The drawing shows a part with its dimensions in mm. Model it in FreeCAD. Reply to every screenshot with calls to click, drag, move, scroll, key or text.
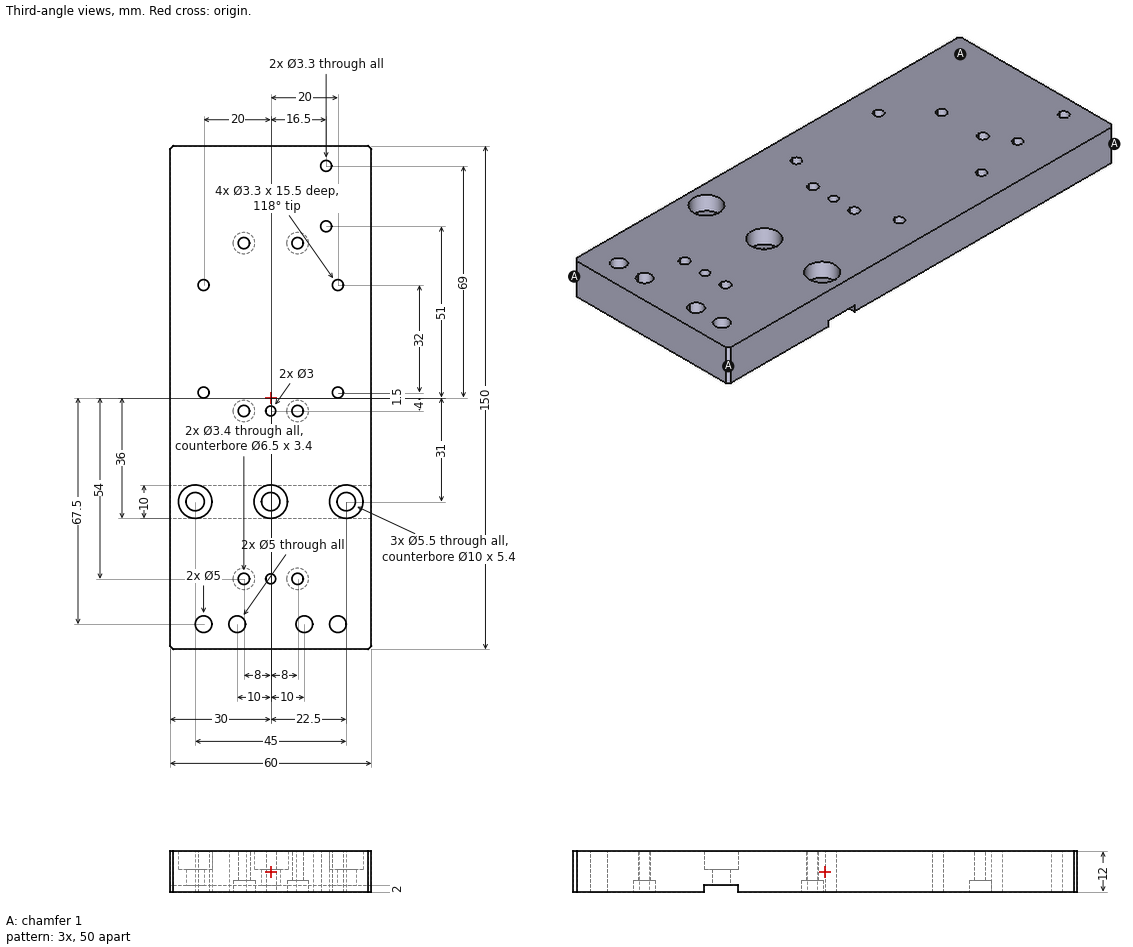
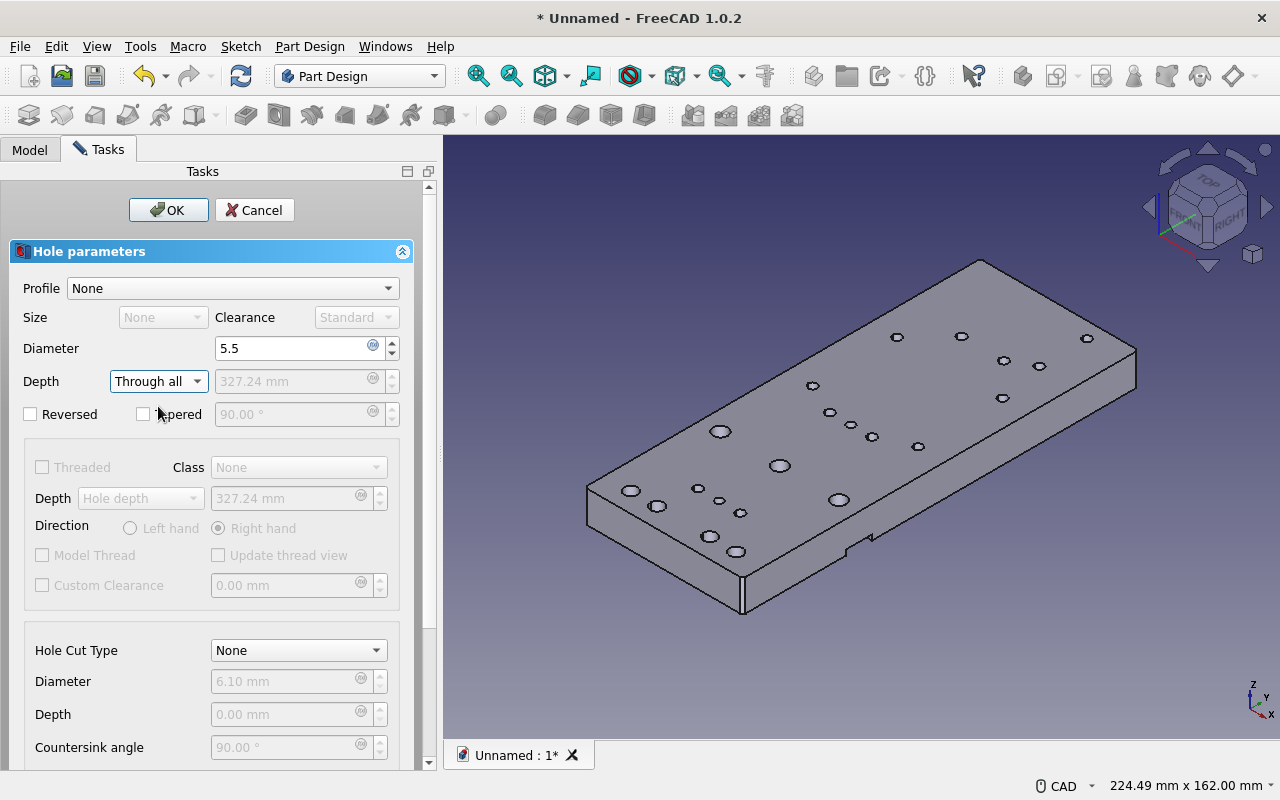
click(300, 650)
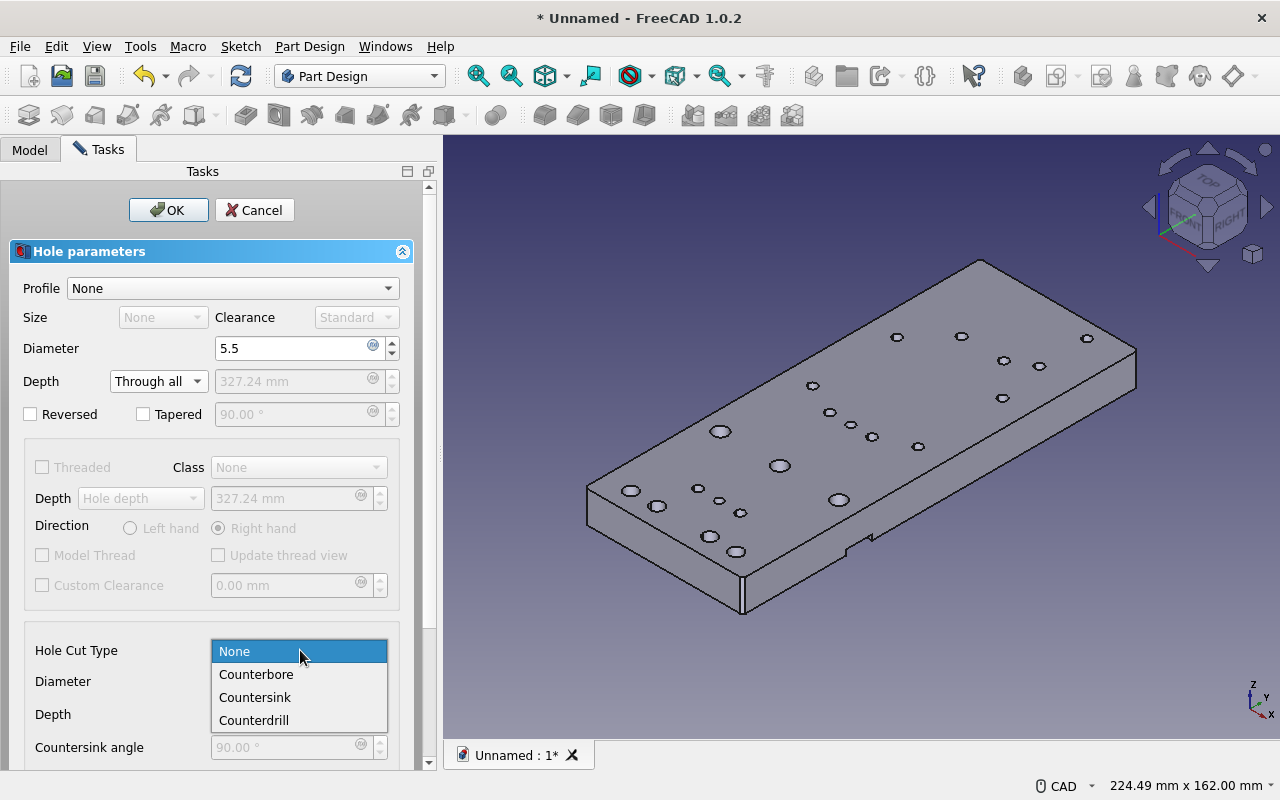
click(298, 674)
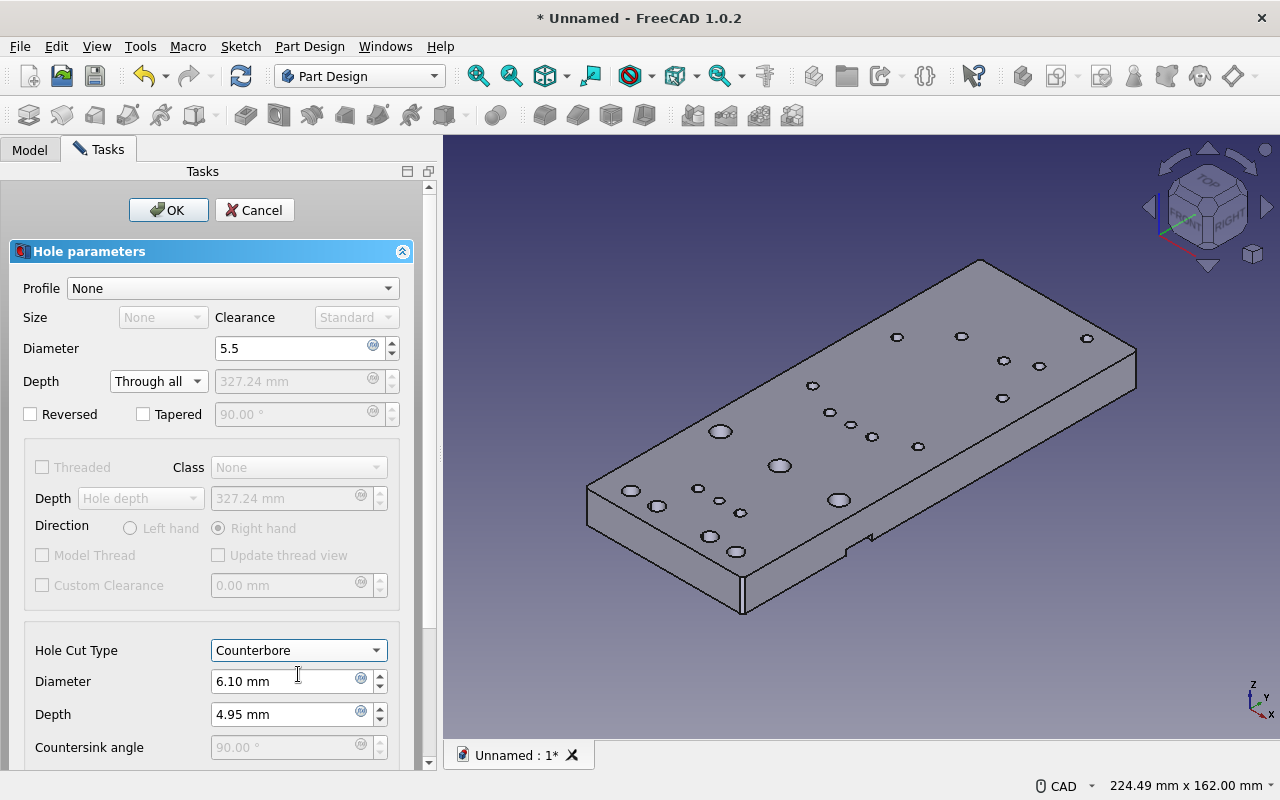
triple_click(292, 682)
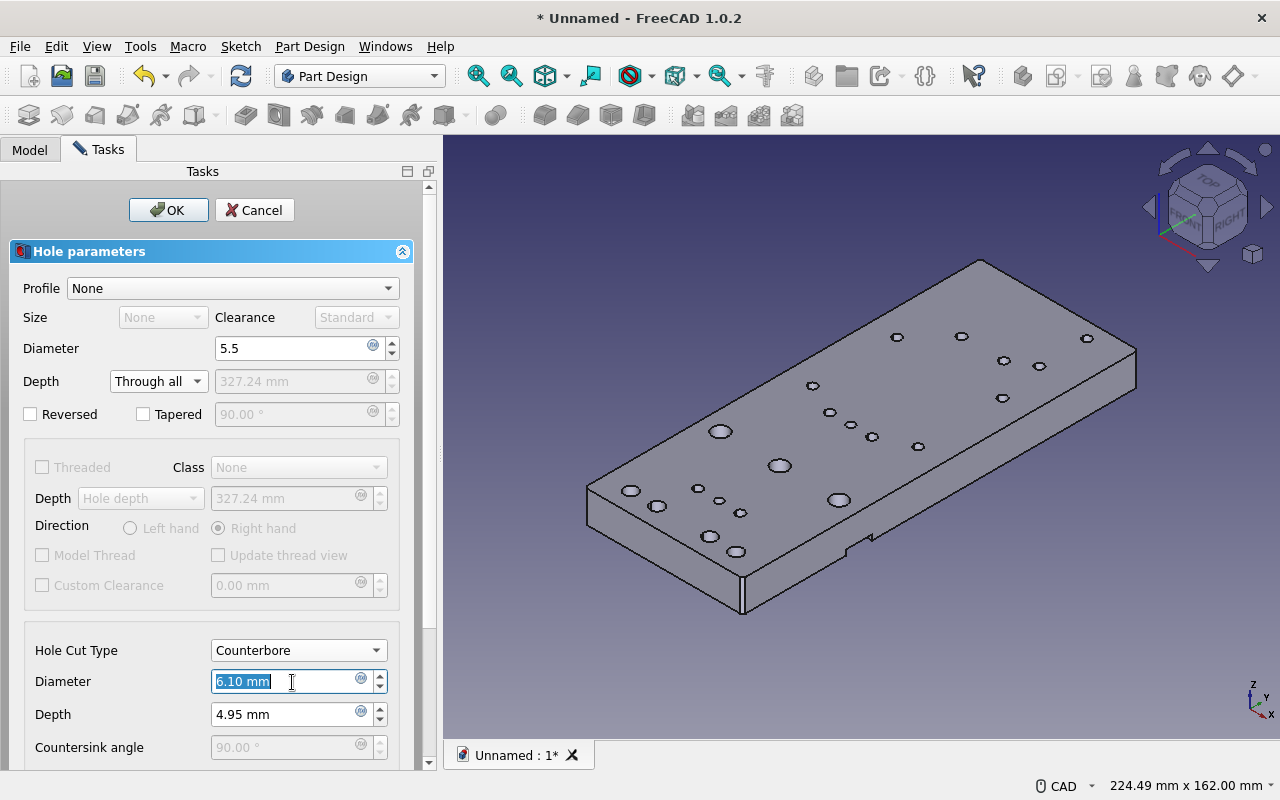
text(10)
key(Tab)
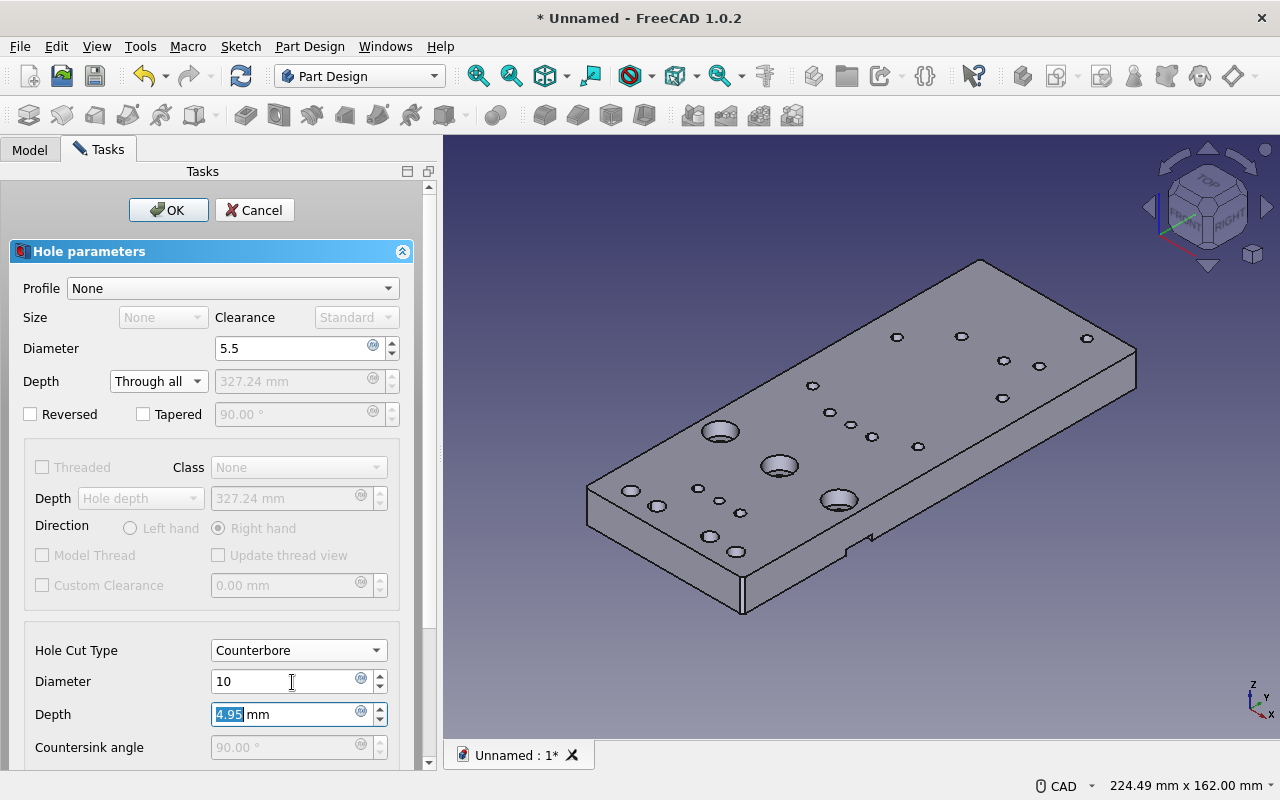
text(5.4)
key(Tab)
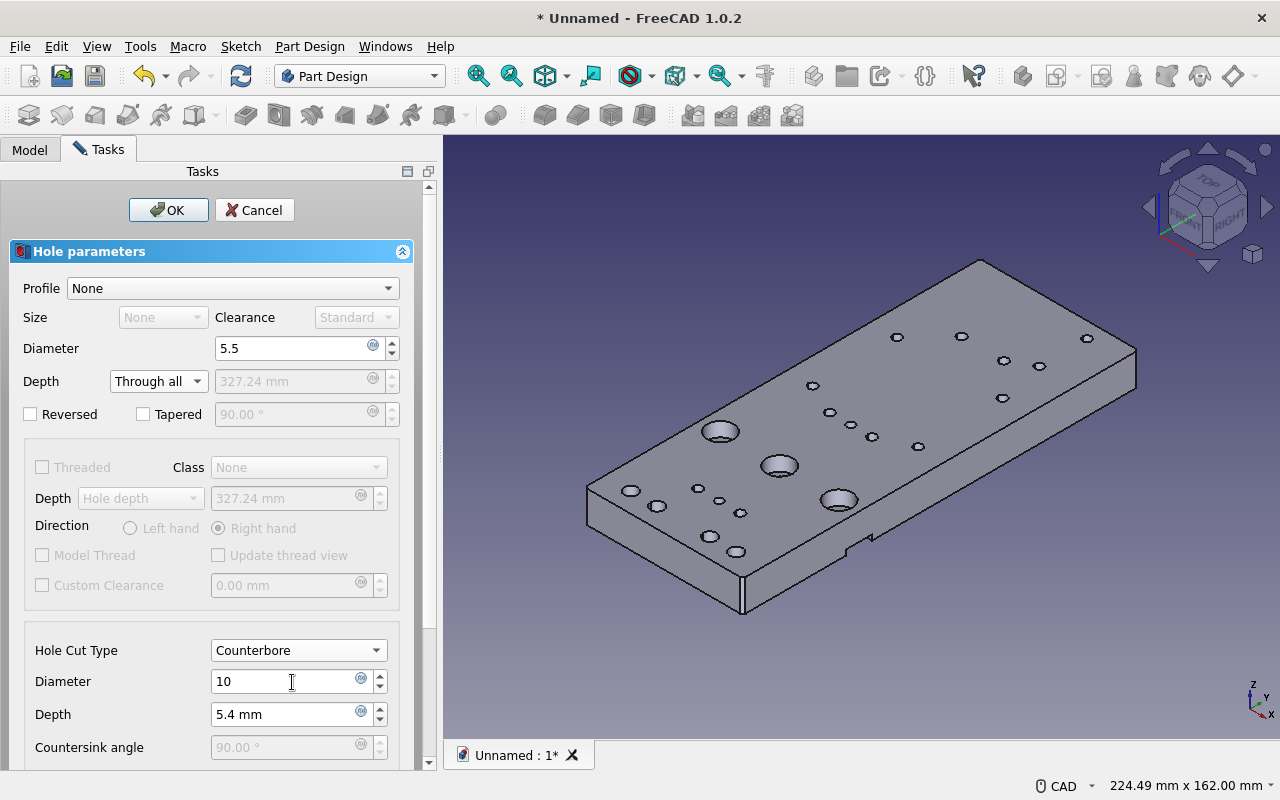
click(169, 210)